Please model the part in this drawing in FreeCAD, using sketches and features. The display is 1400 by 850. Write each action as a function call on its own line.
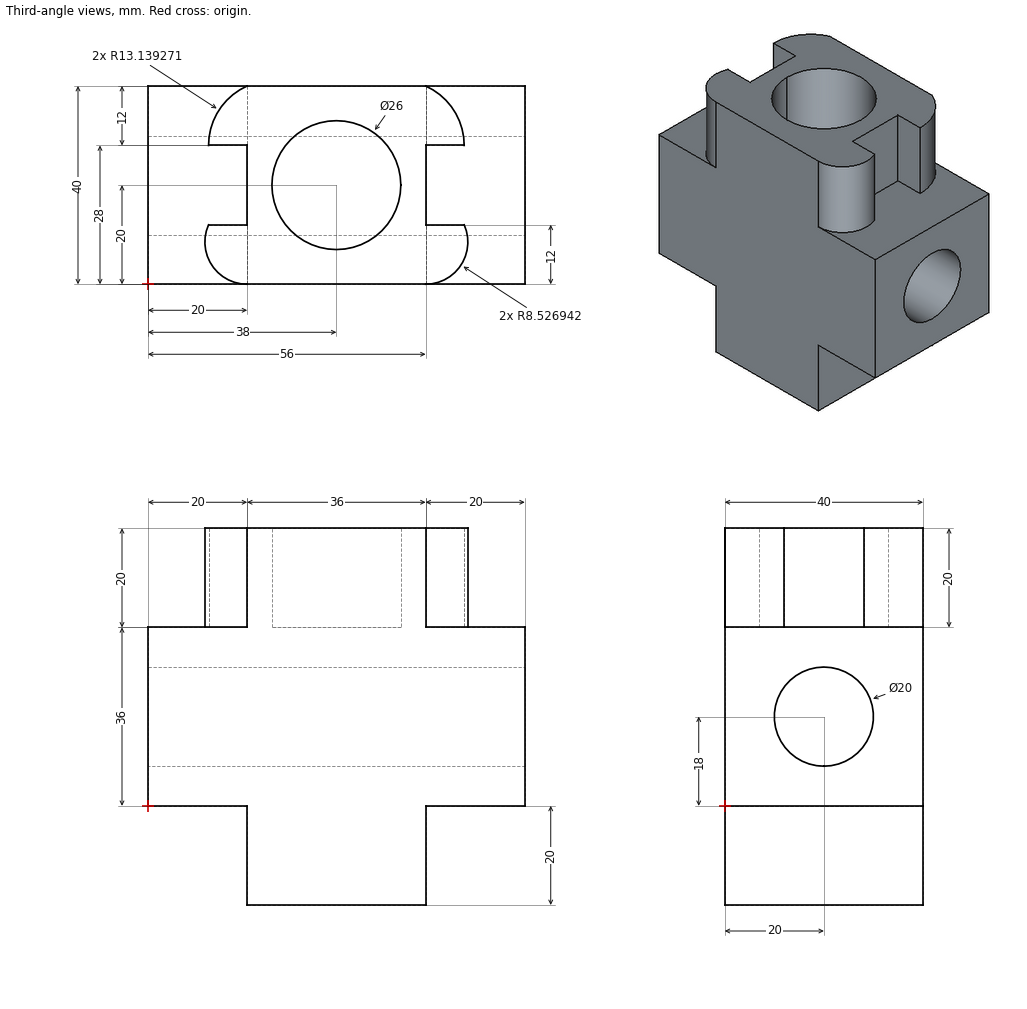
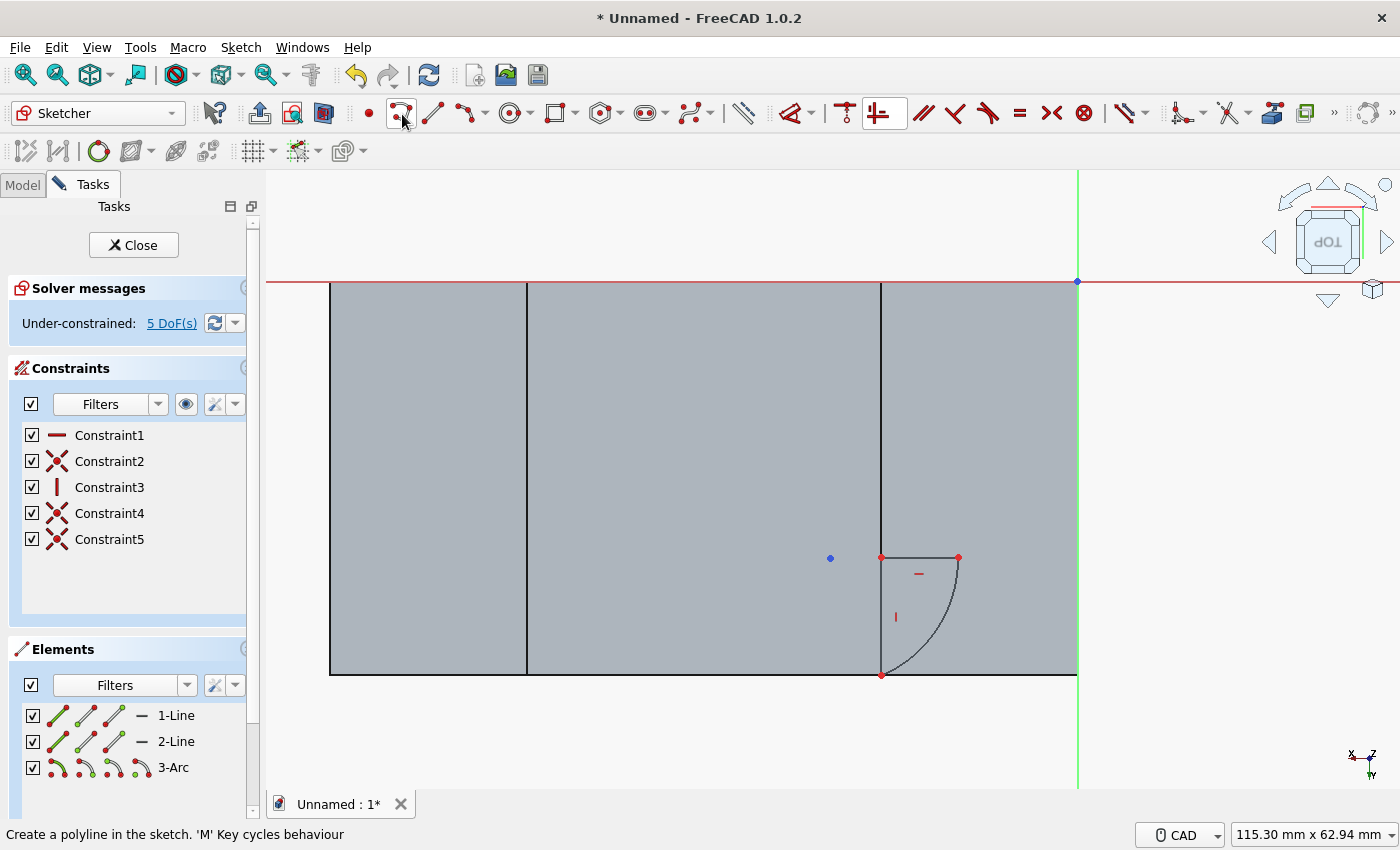
click(527, 675)
click(527, 557)
click(451, 557)
right_click(451, 557)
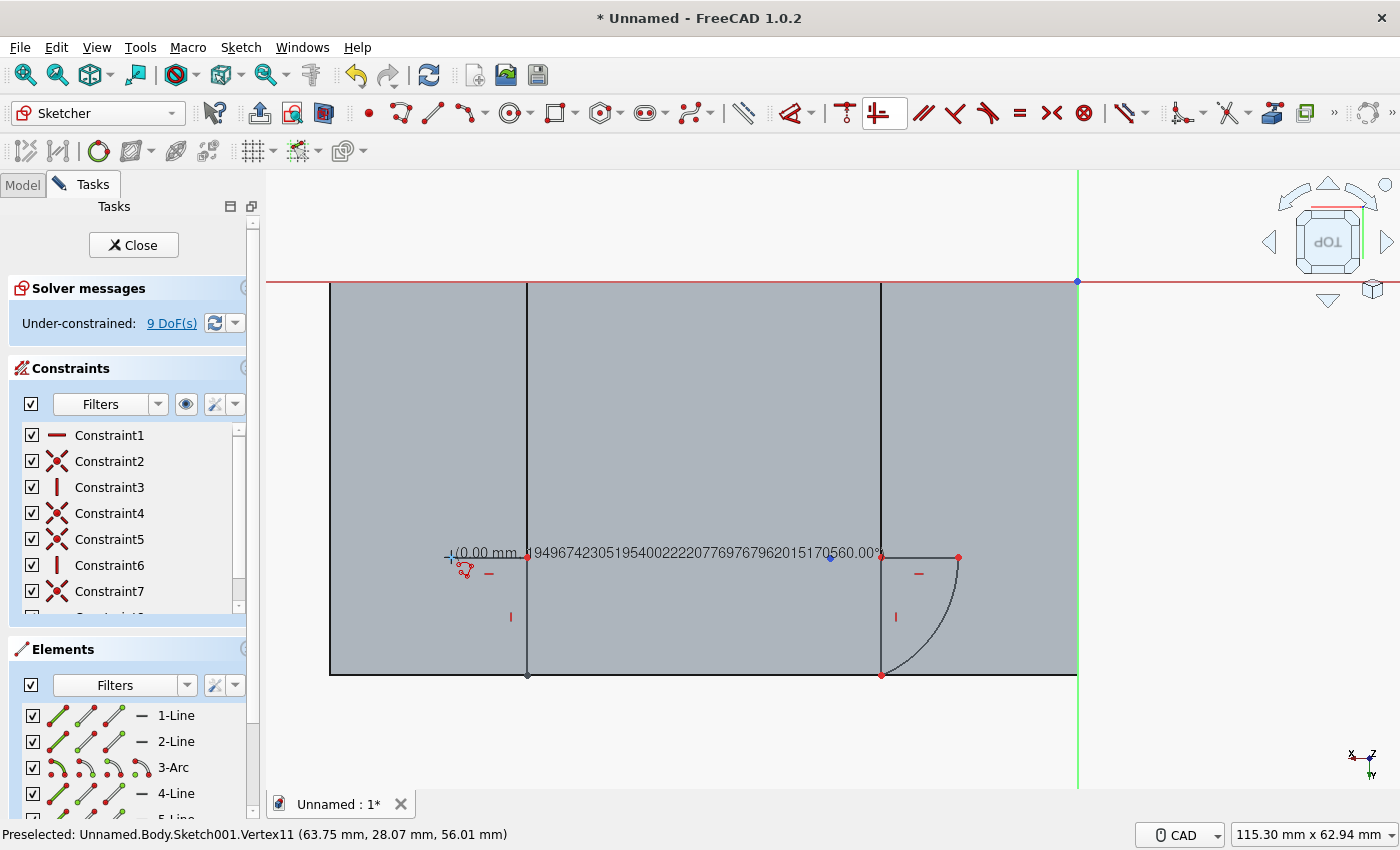
click(466, 114)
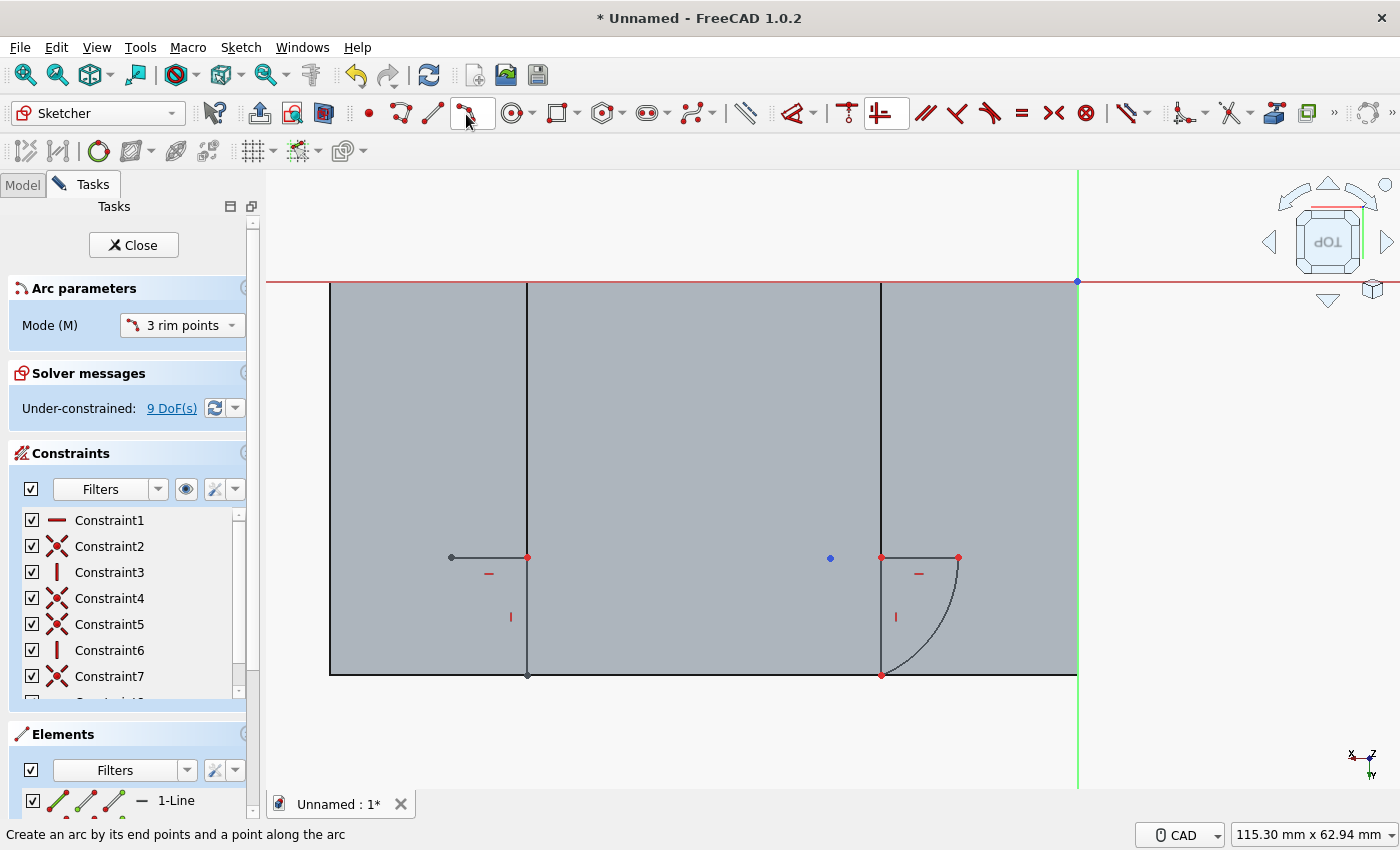
click(451, 558)
click(527, 676)
click(471, 628)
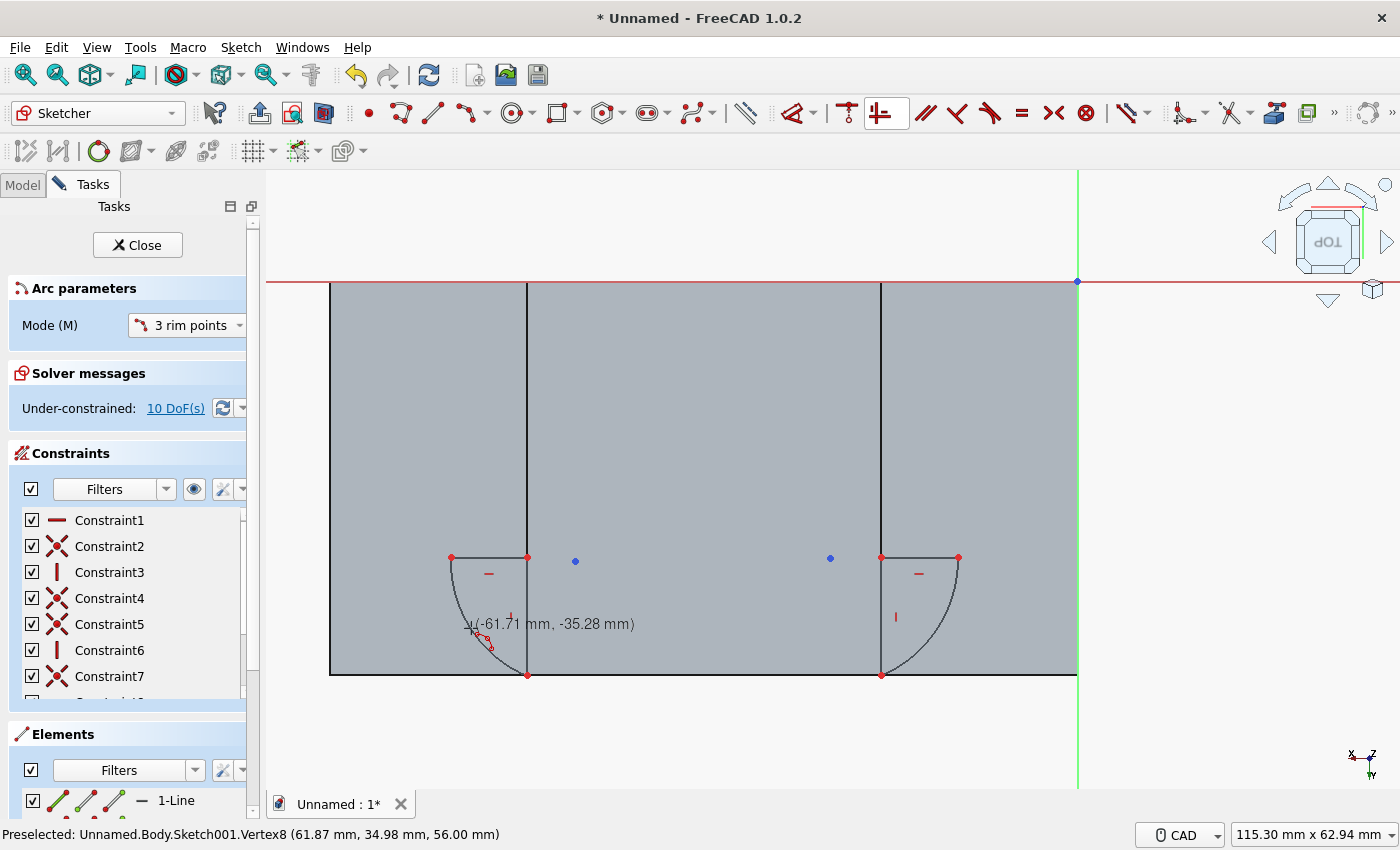
click(402, 114)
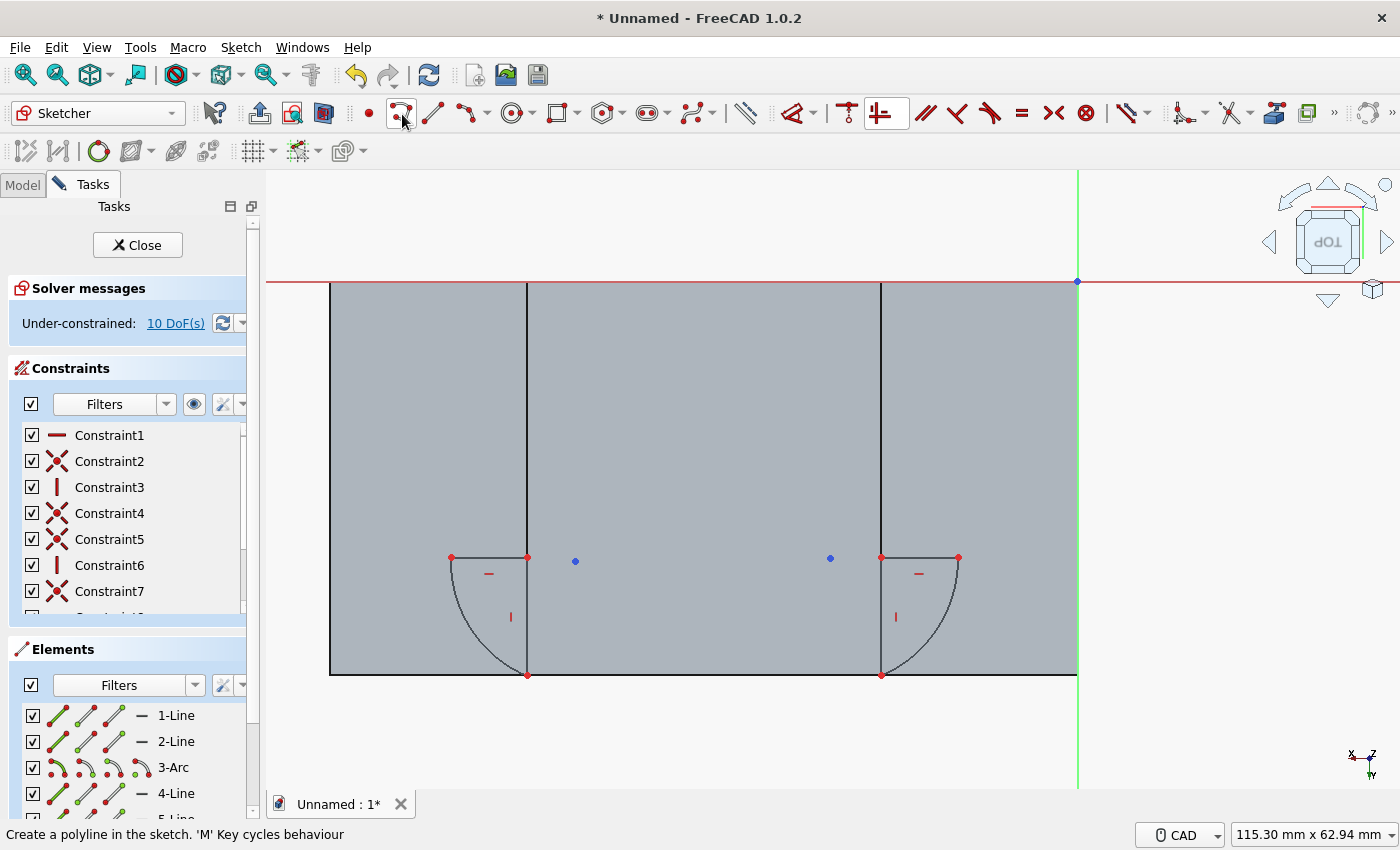
click(451, 400)
click(527, 400)
click(527, 282)
right_click(527, 282)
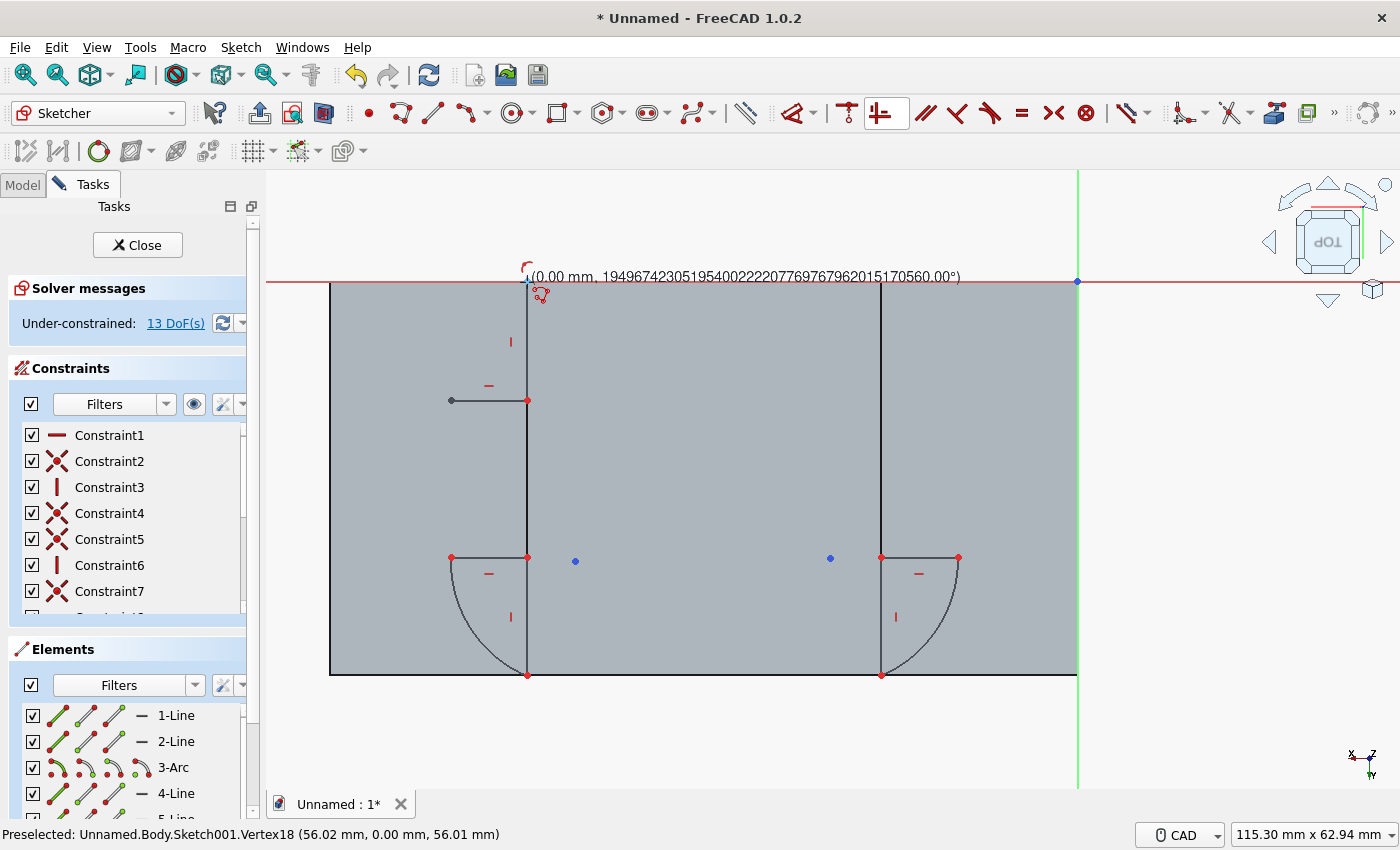
click(466, 114)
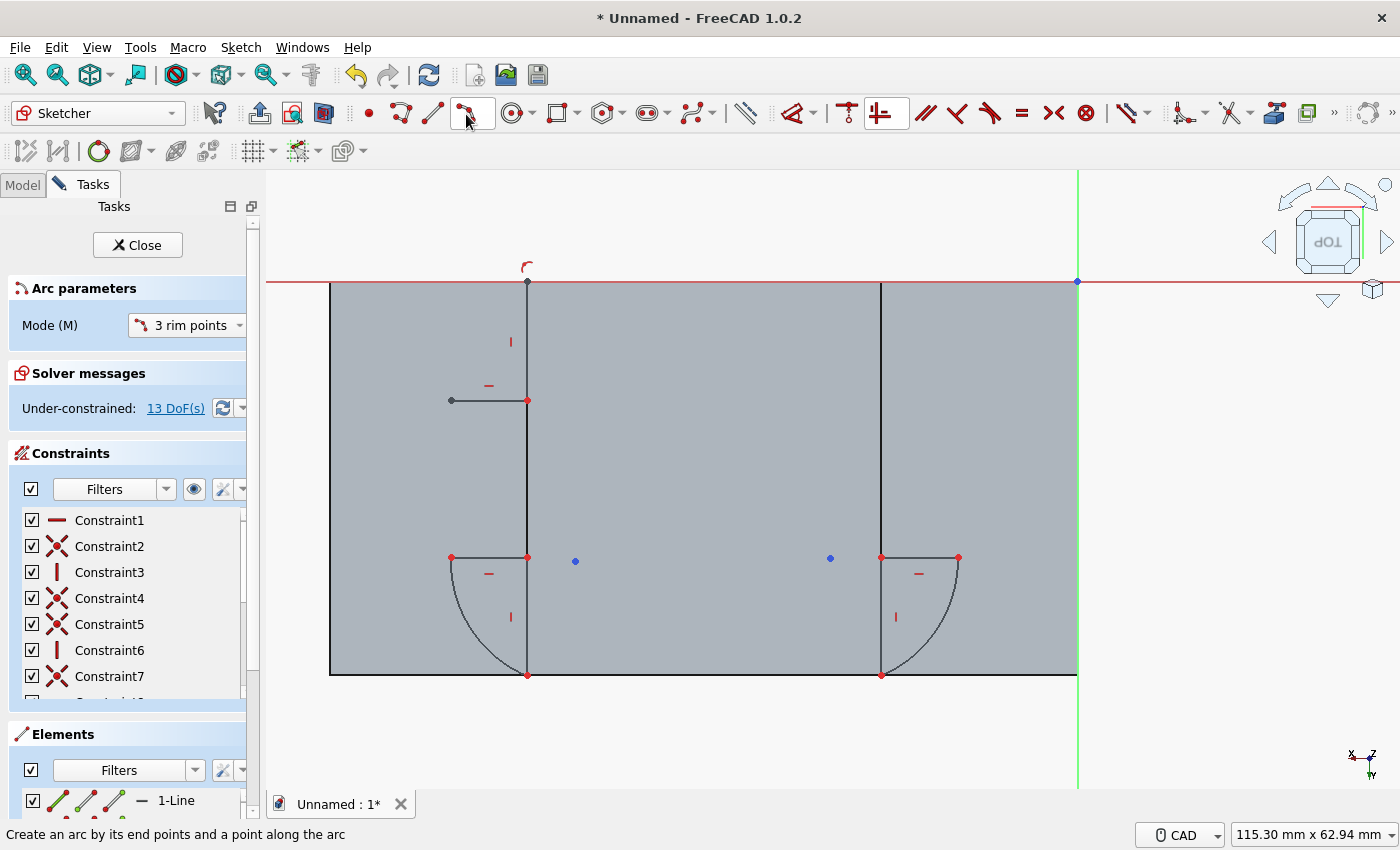
click(527, 282)
click(451, 401)
click(457, 320)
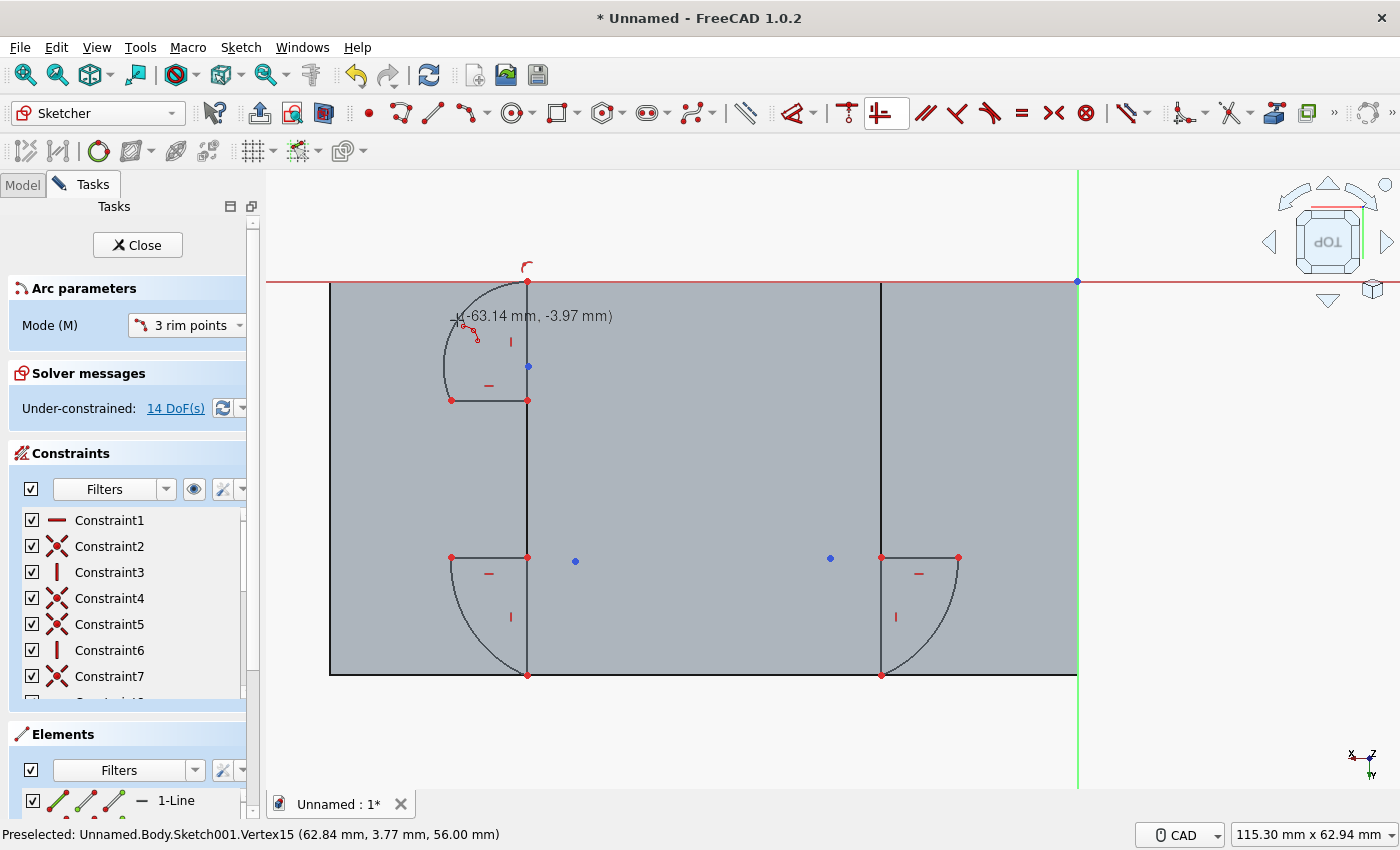
click(402, 114)